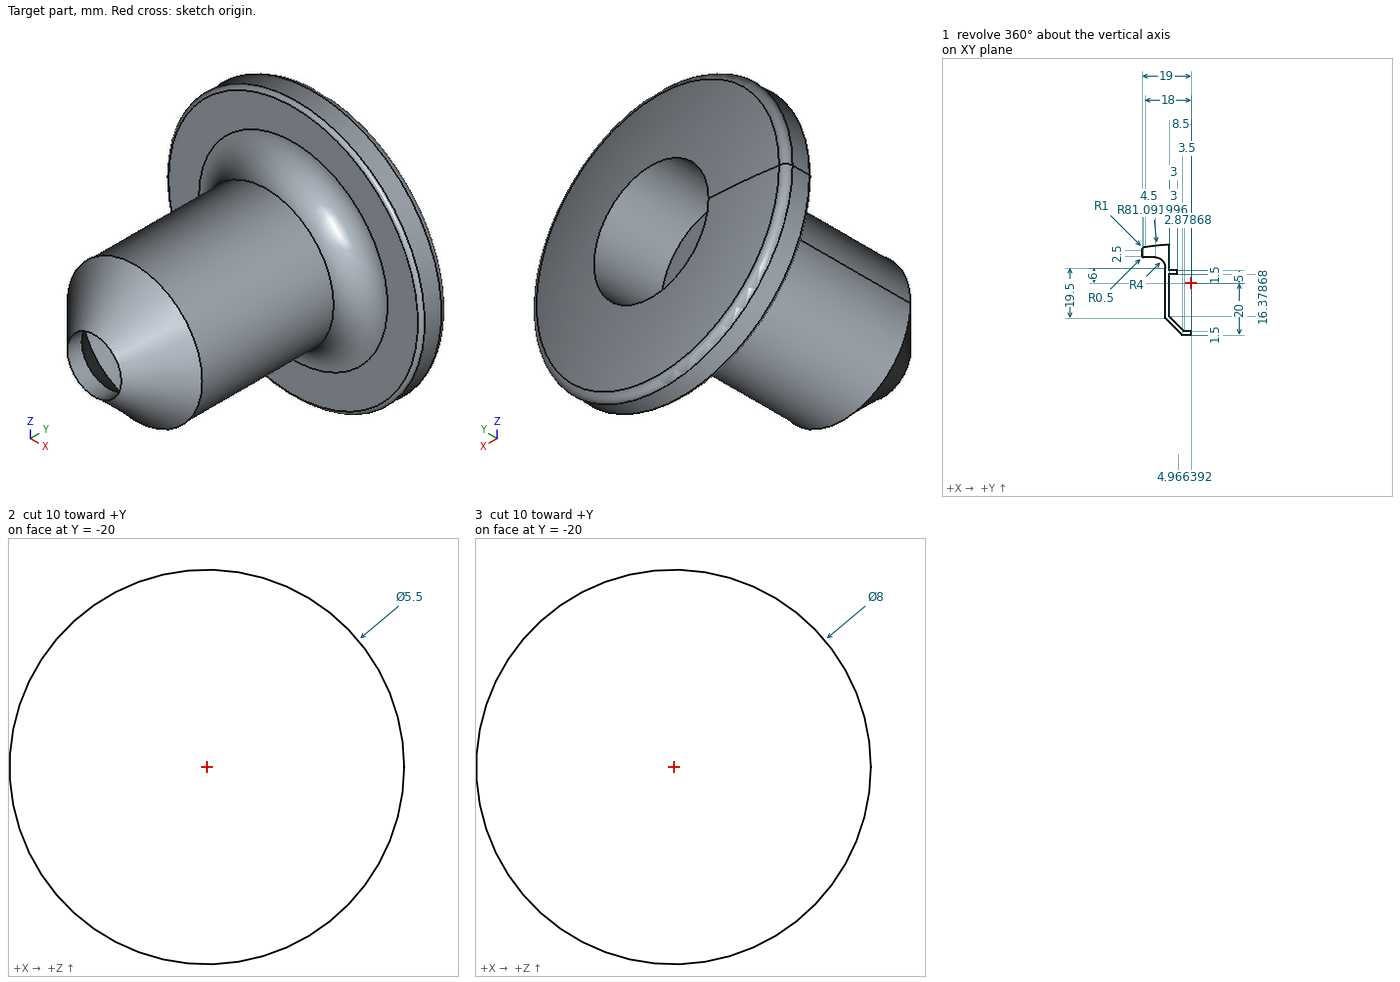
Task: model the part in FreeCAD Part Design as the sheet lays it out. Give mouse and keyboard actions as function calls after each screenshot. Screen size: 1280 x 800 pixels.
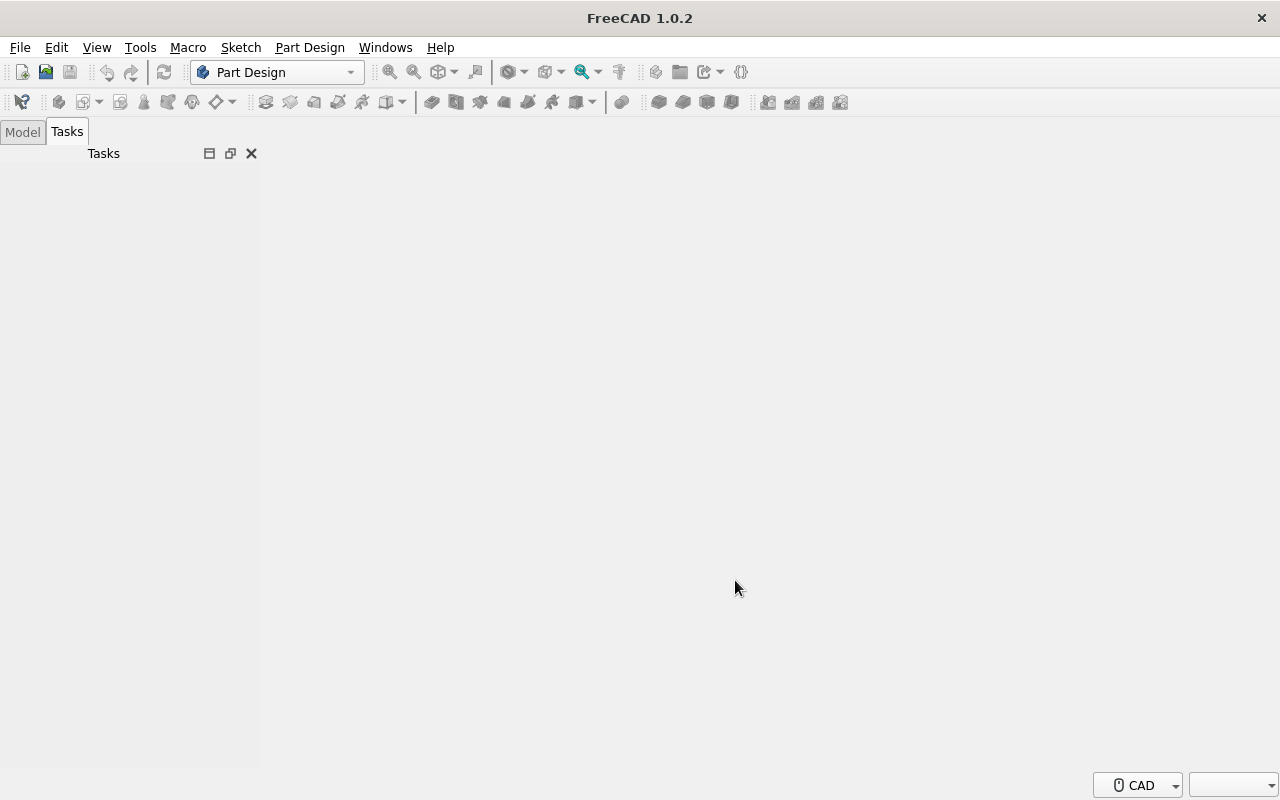
click(22, 72)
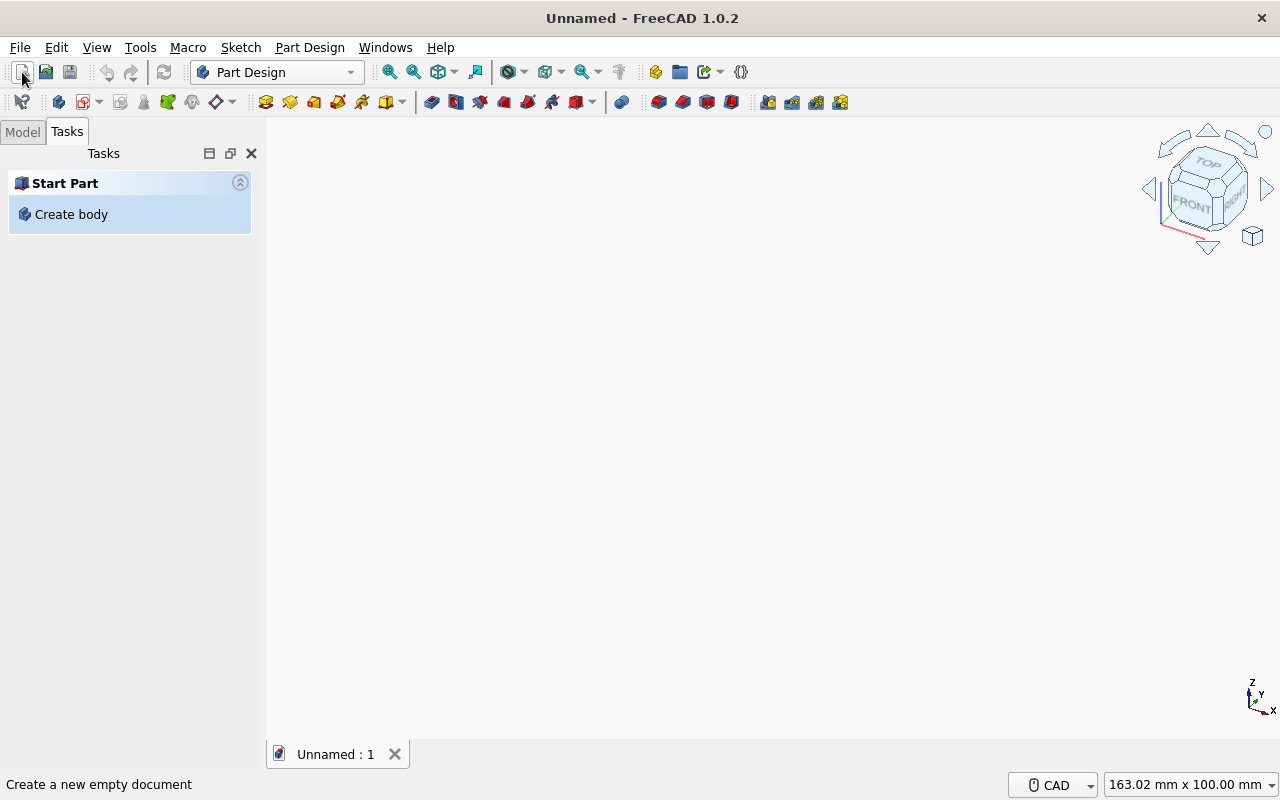
click(84, 102)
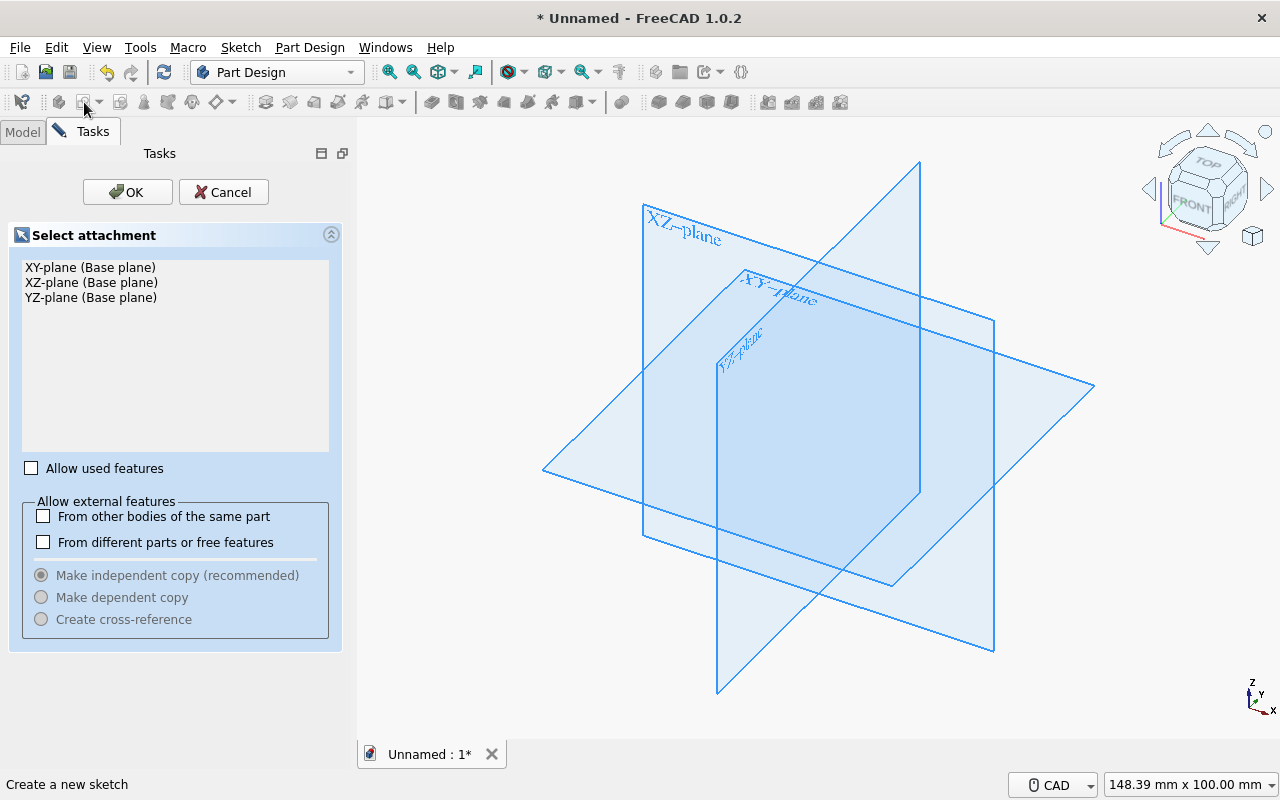
click(82, 268)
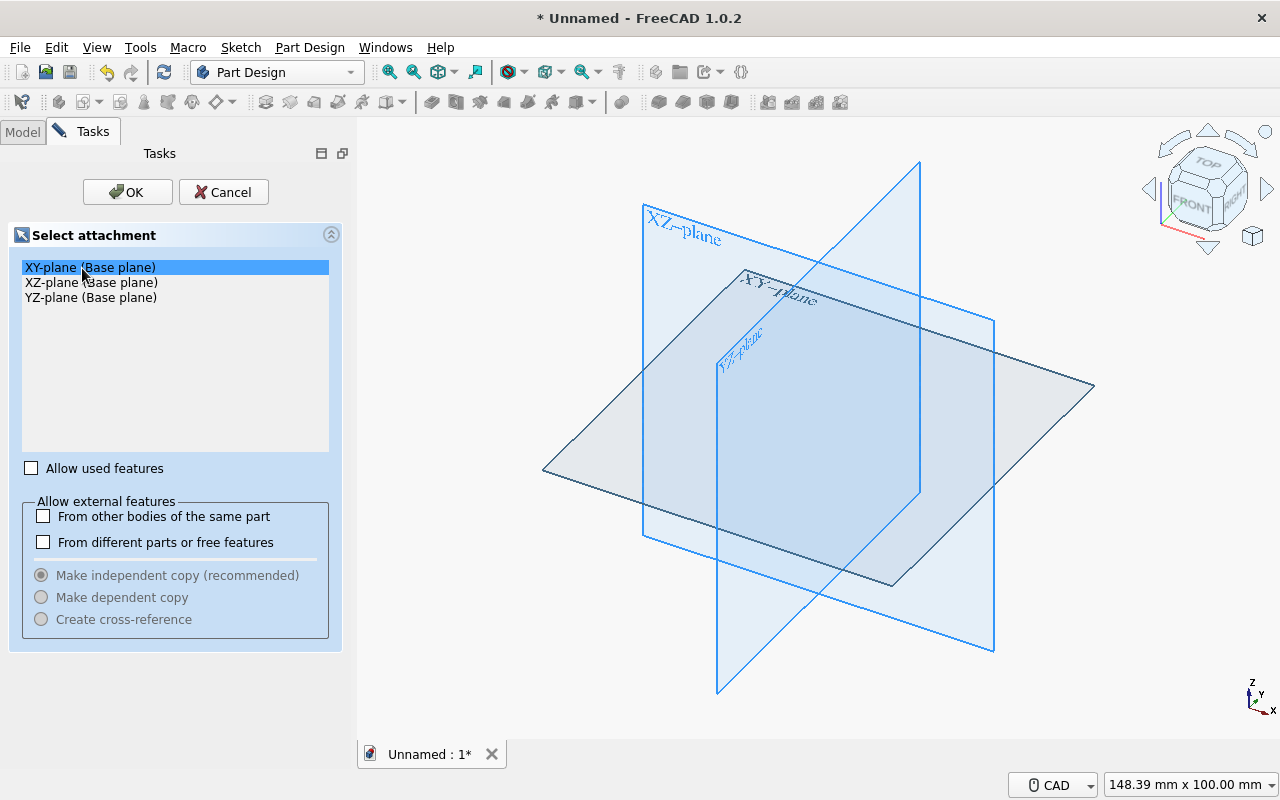
click(128, 192)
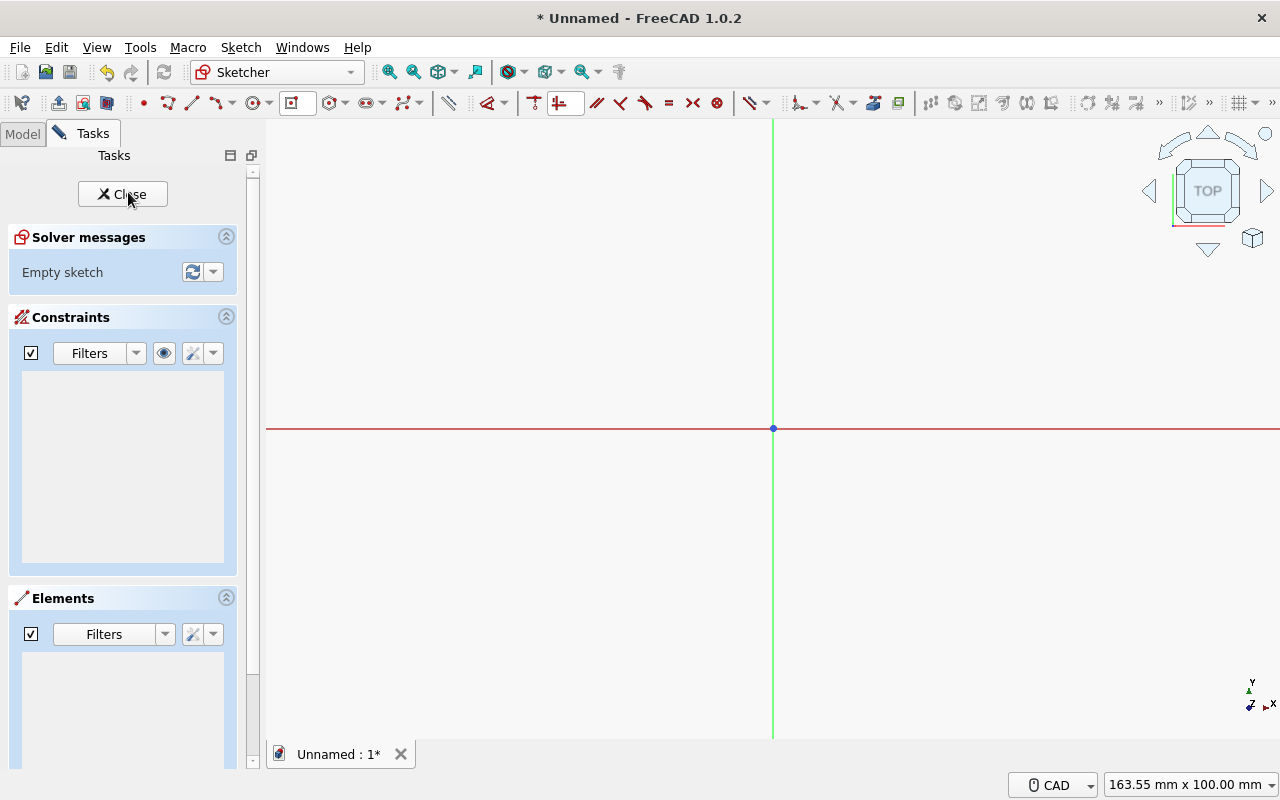
scroll(726, 464, up, 3)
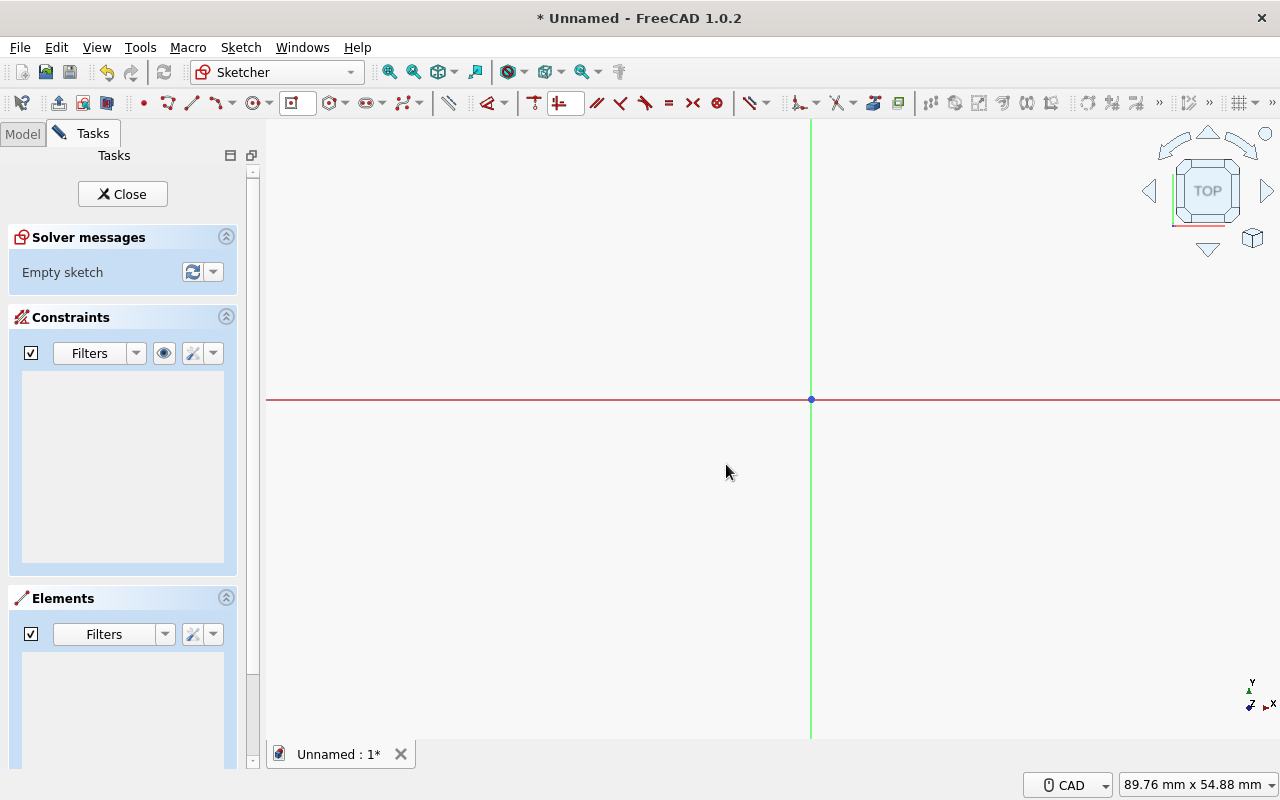
click(192, 104)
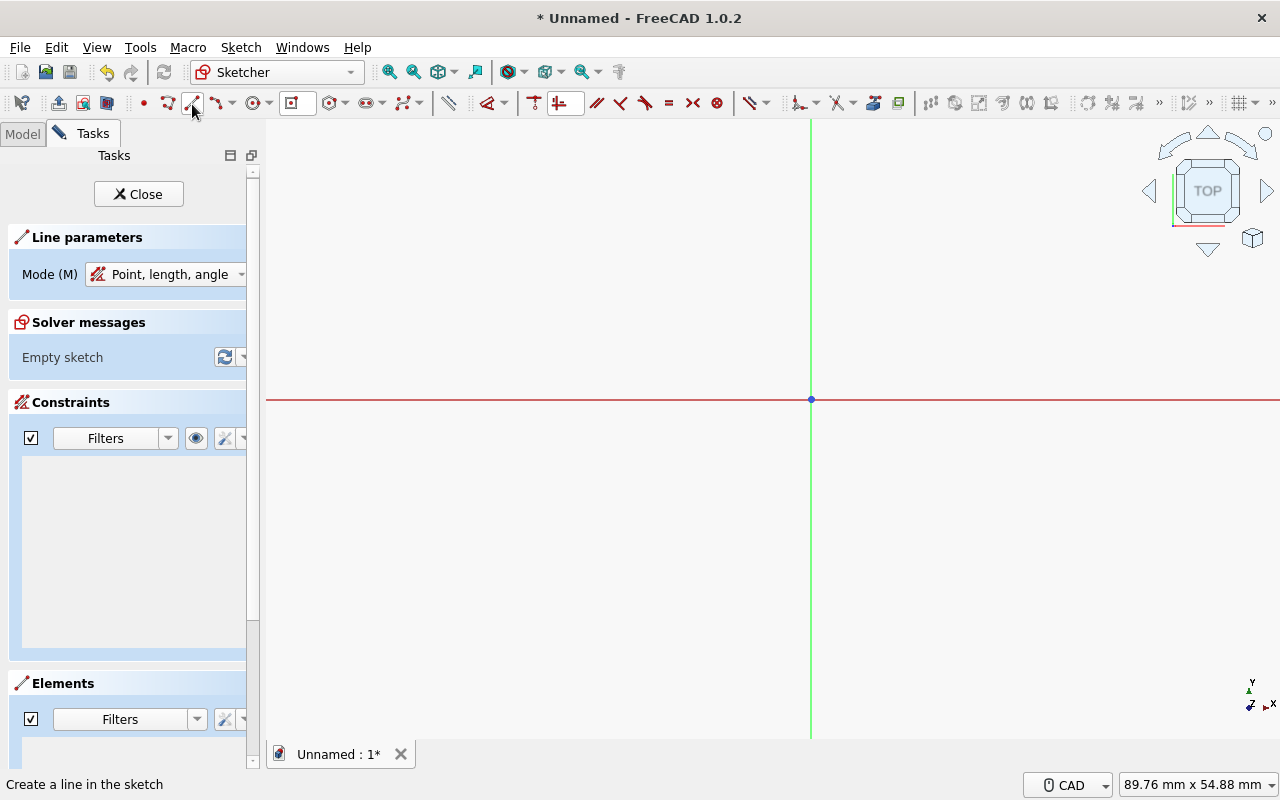
click(597, 253)
click(597, 281)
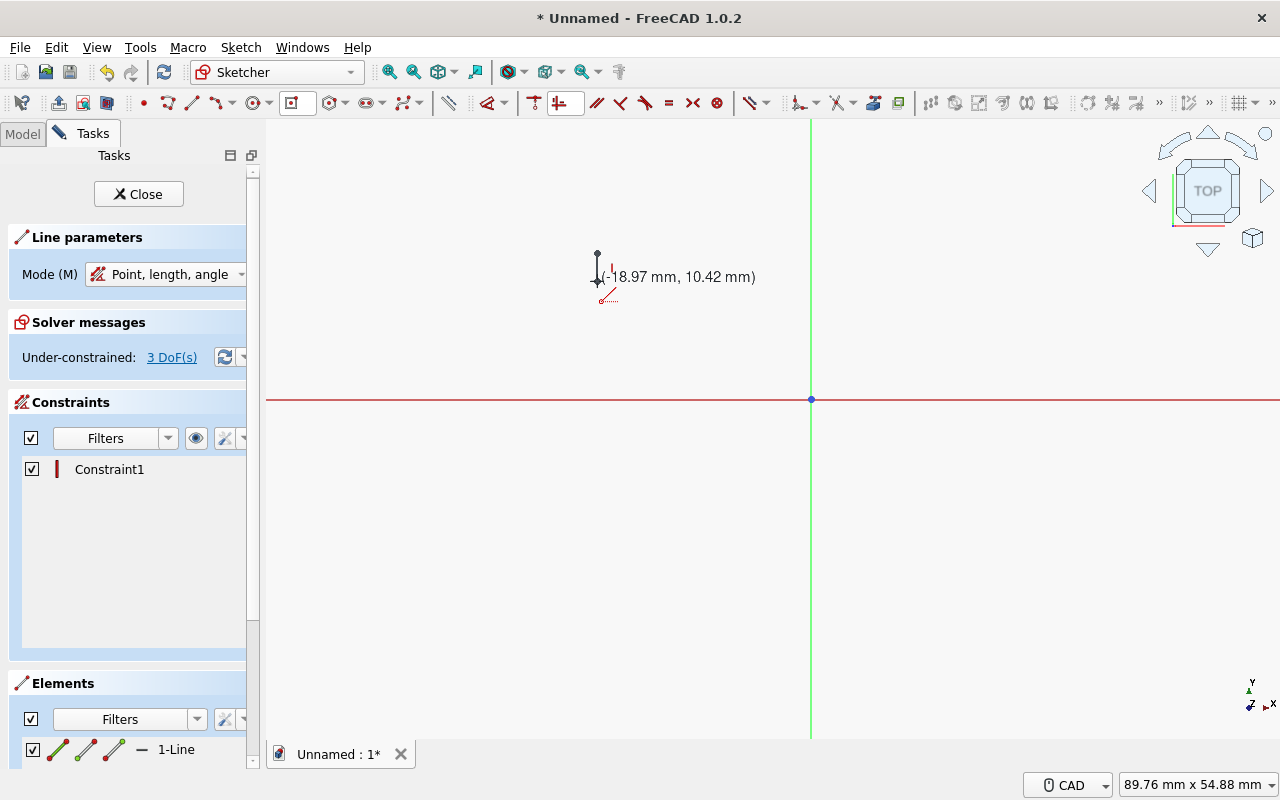
scroll(602, 287, up, 4)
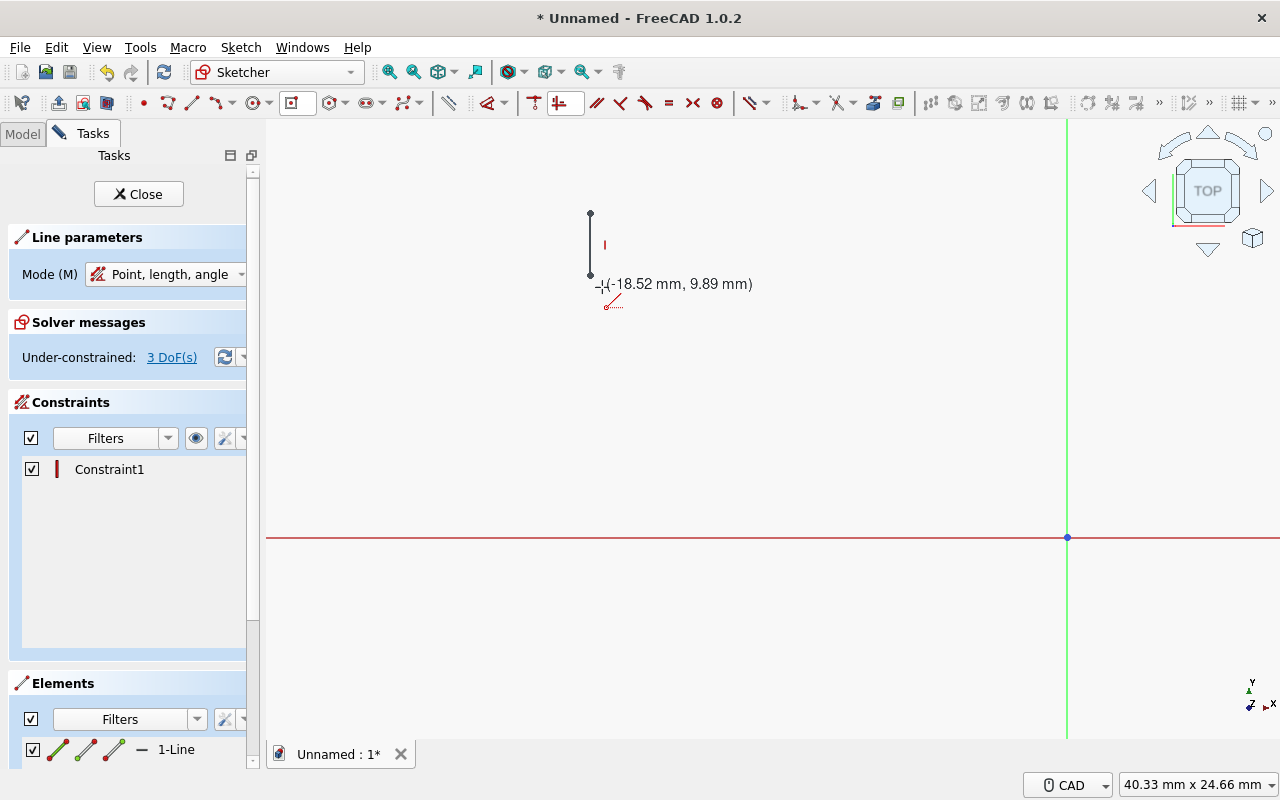
click(602, 286)
click(715, 286)